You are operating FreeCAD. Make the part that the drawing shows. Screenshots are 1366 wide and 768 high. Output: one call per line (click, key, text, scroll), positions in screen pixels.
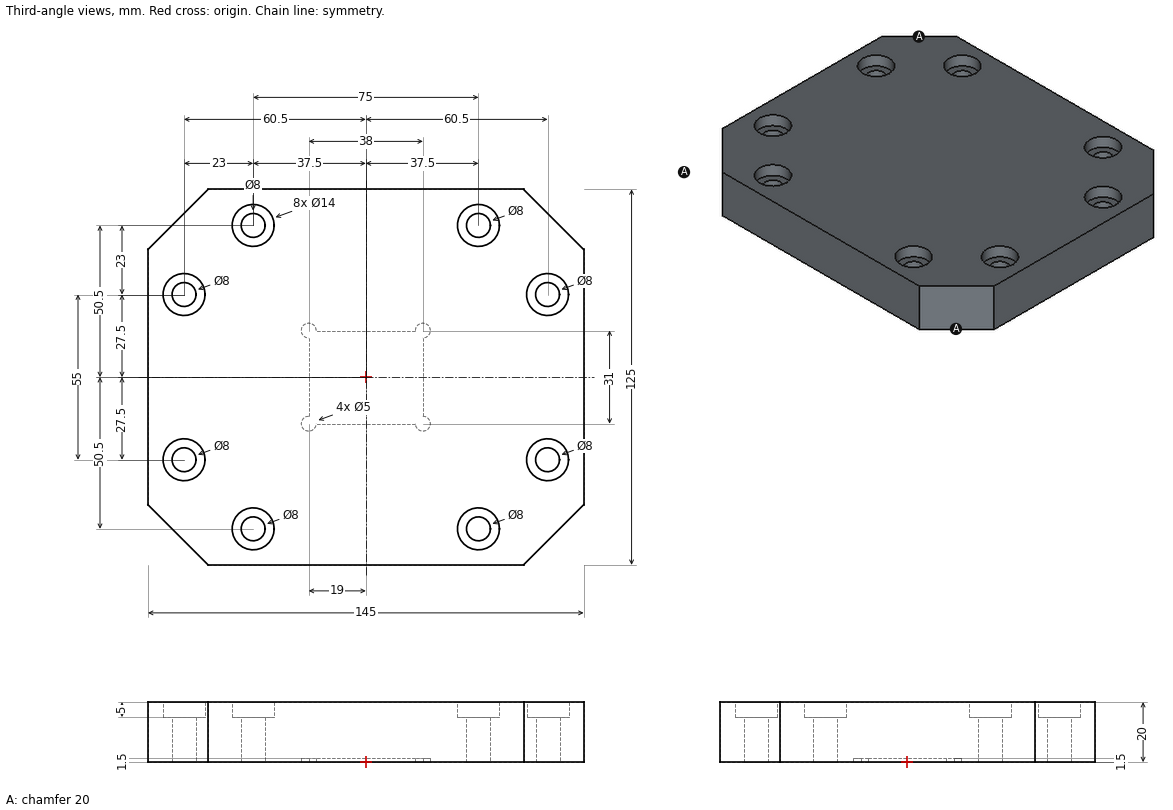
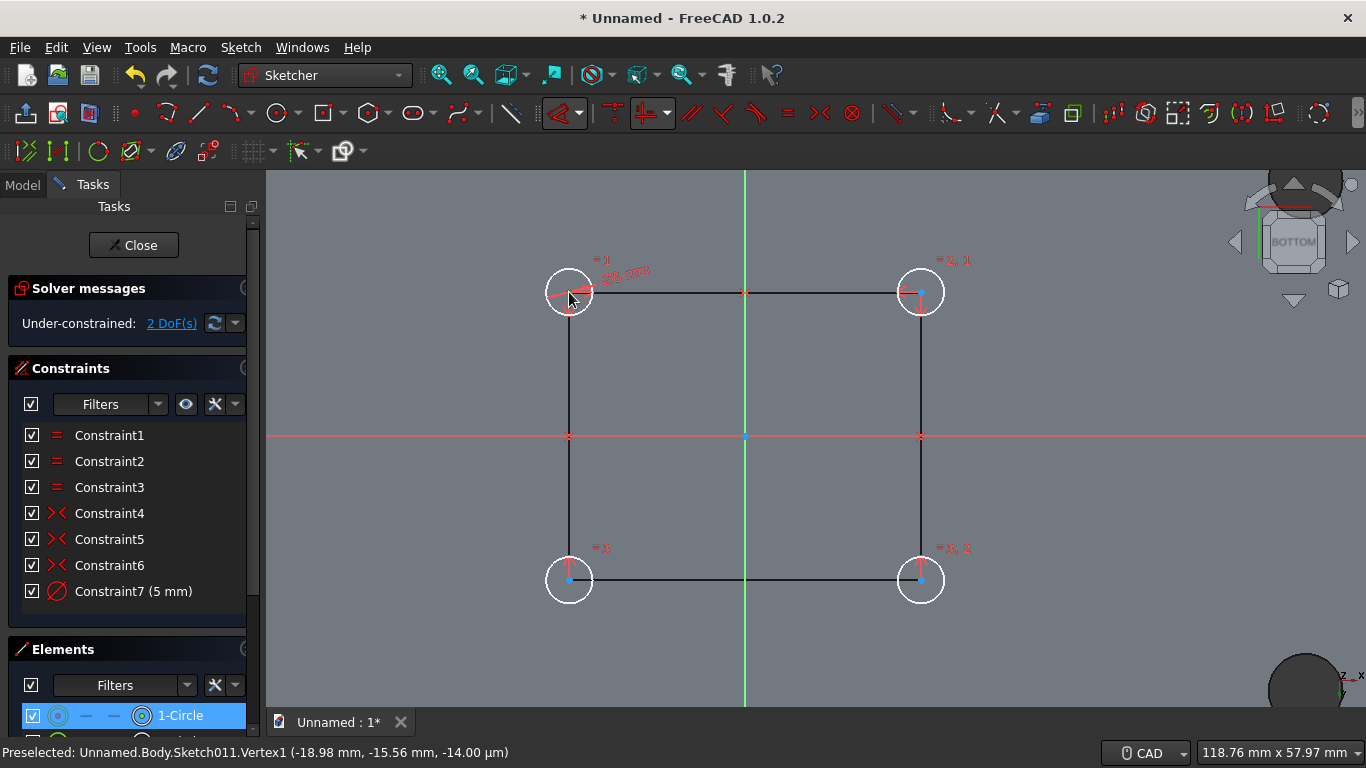
key(l)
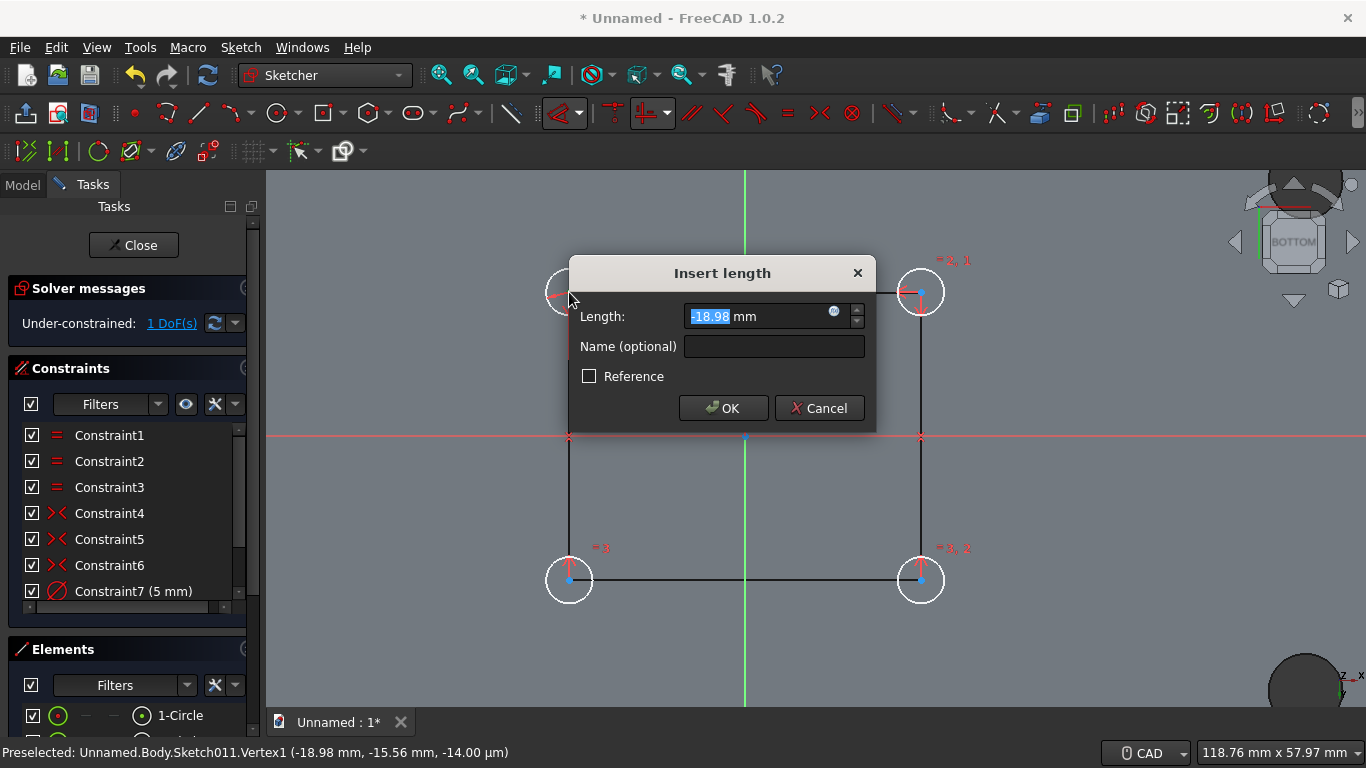
text(-19)
key(Return)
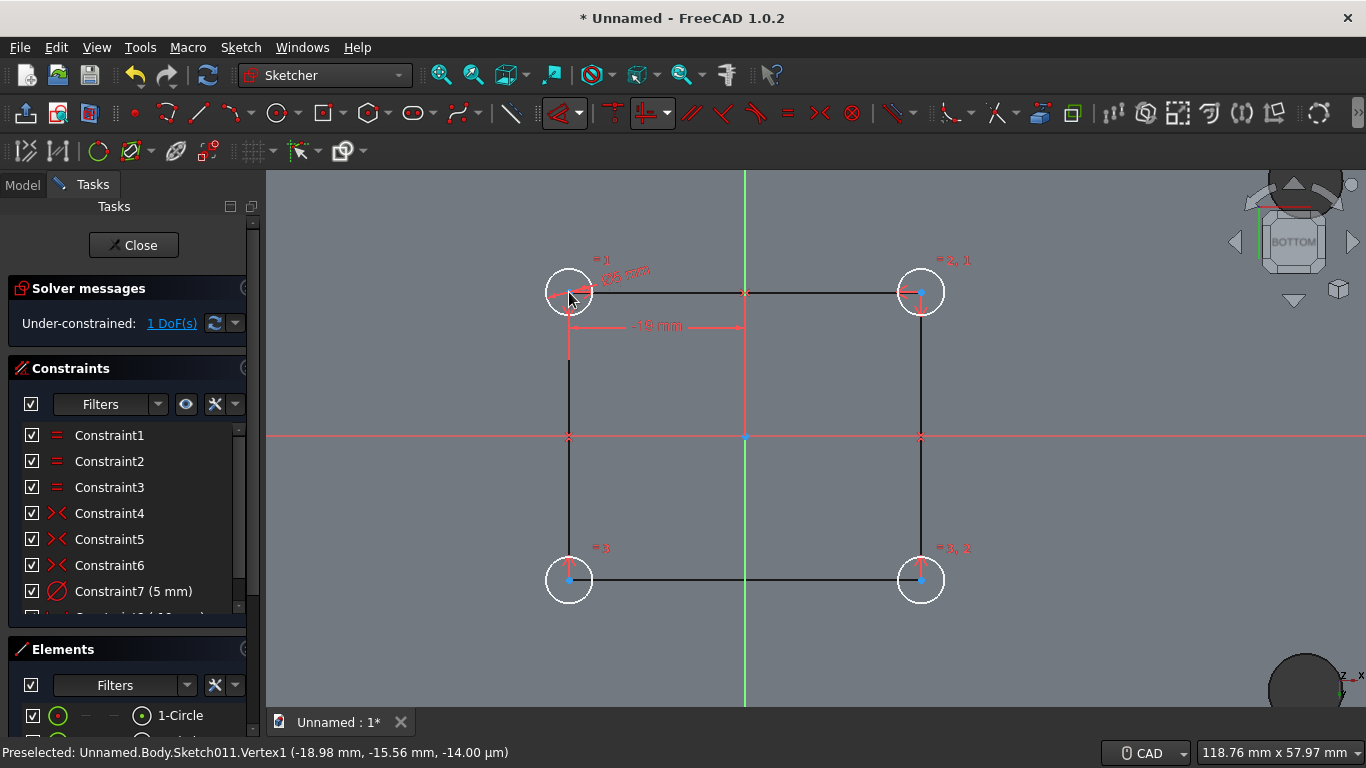
click(921, 292)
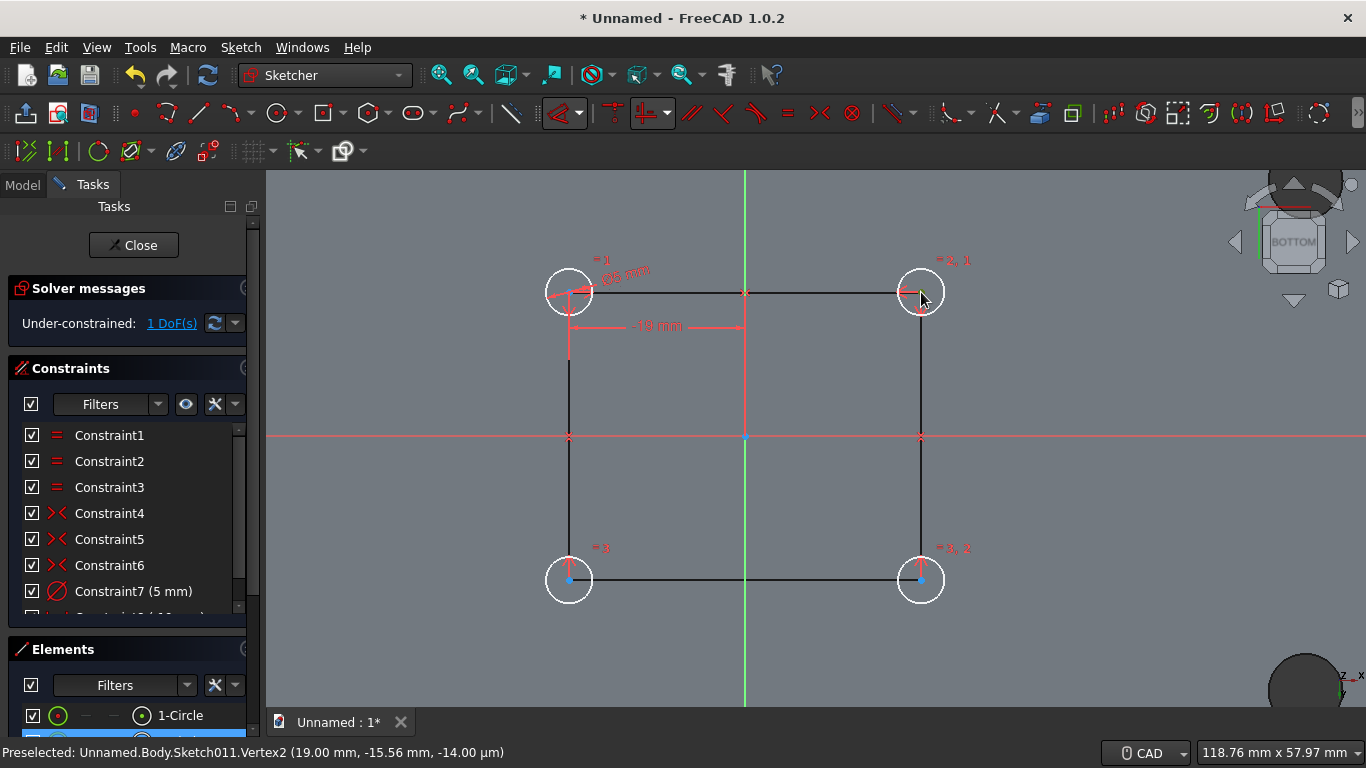
click(921, 580)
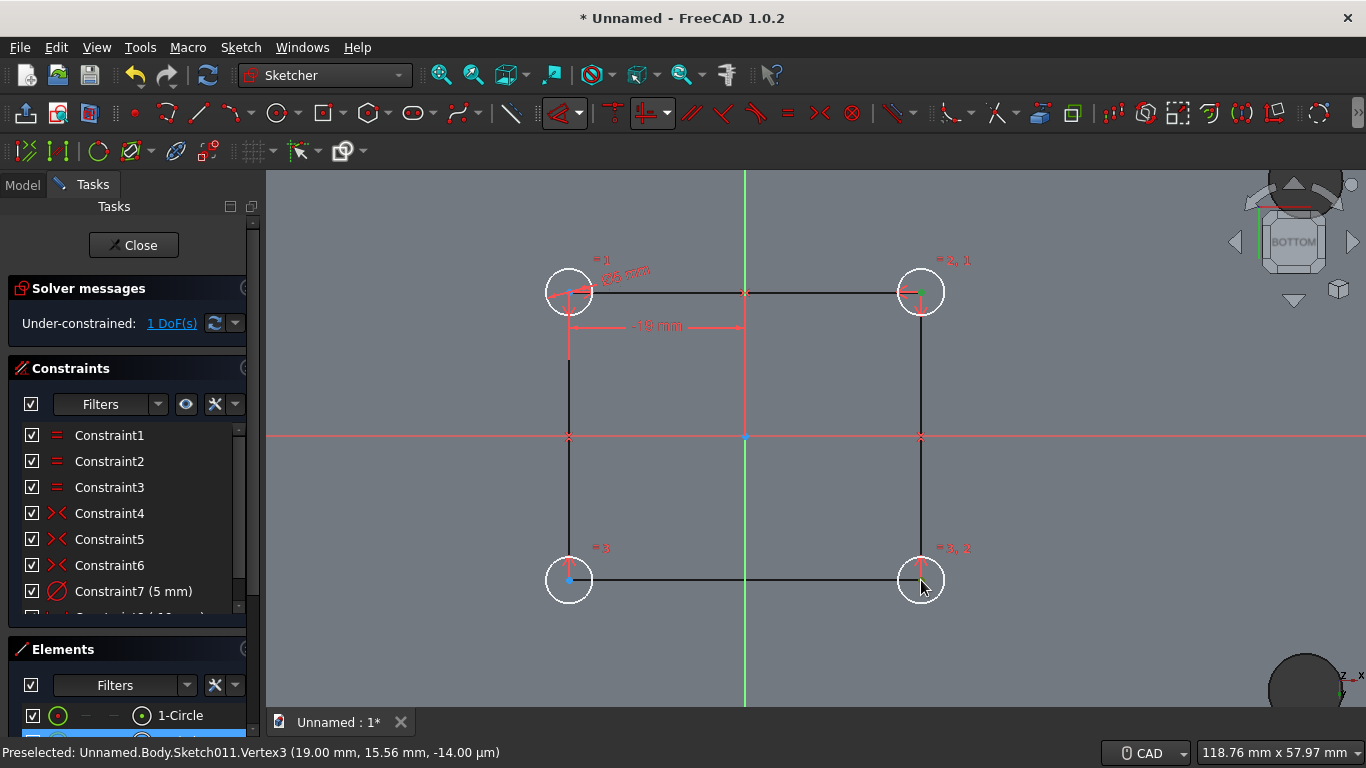
key(i)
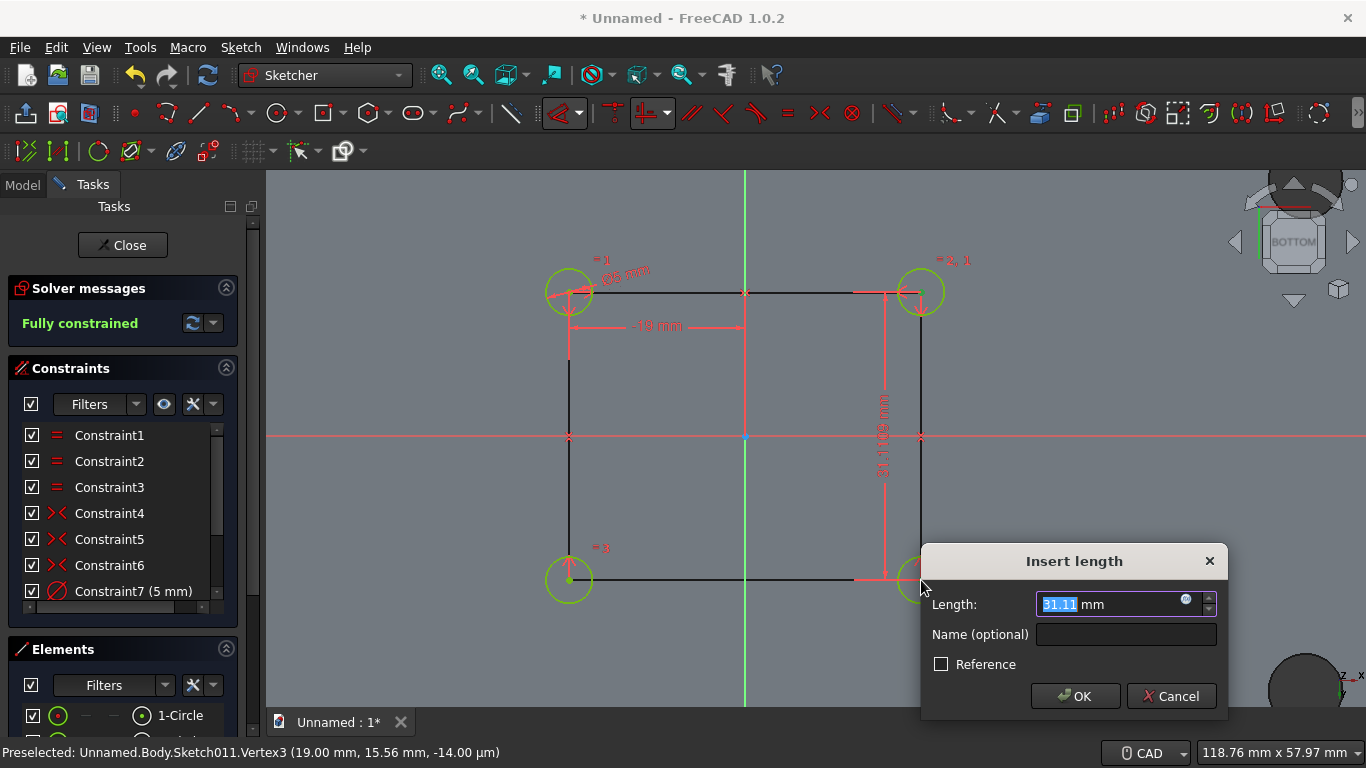
text(31)
key(Return)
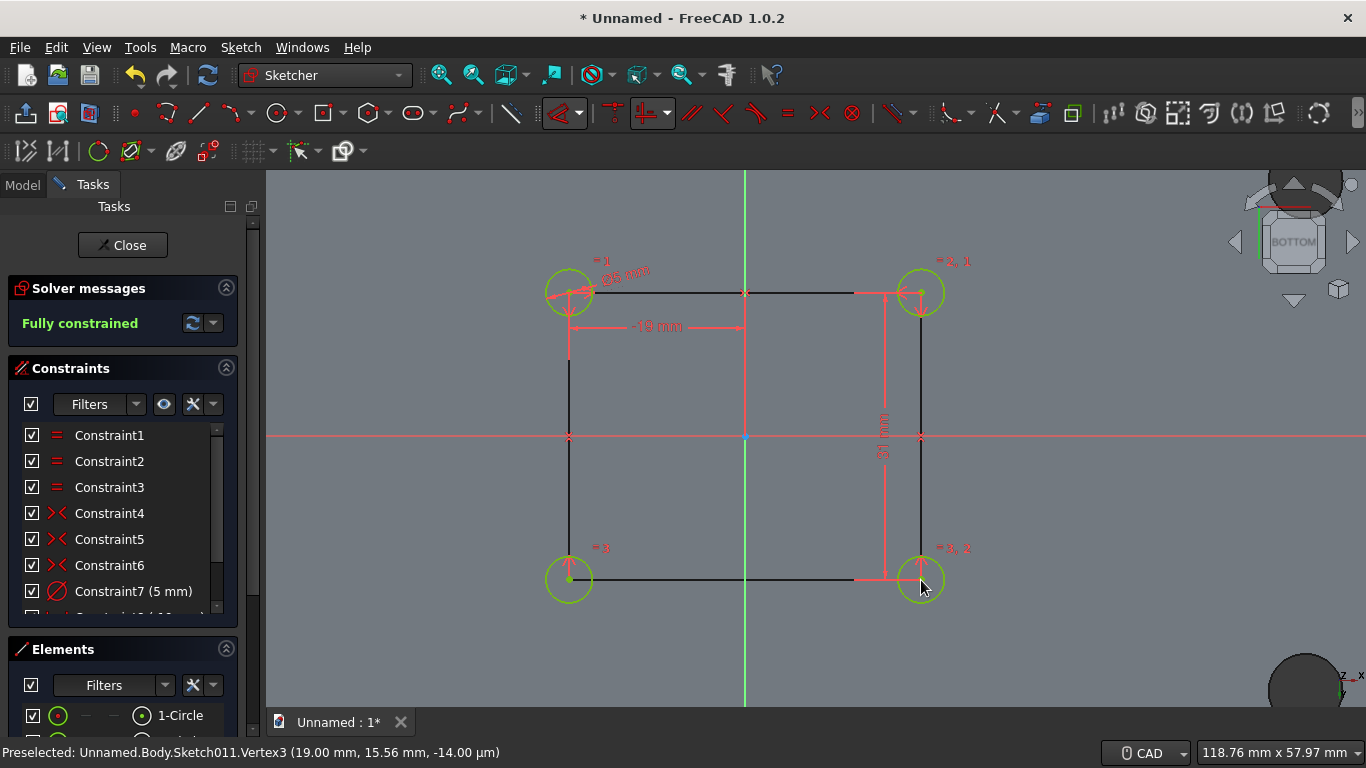
click(123, 245)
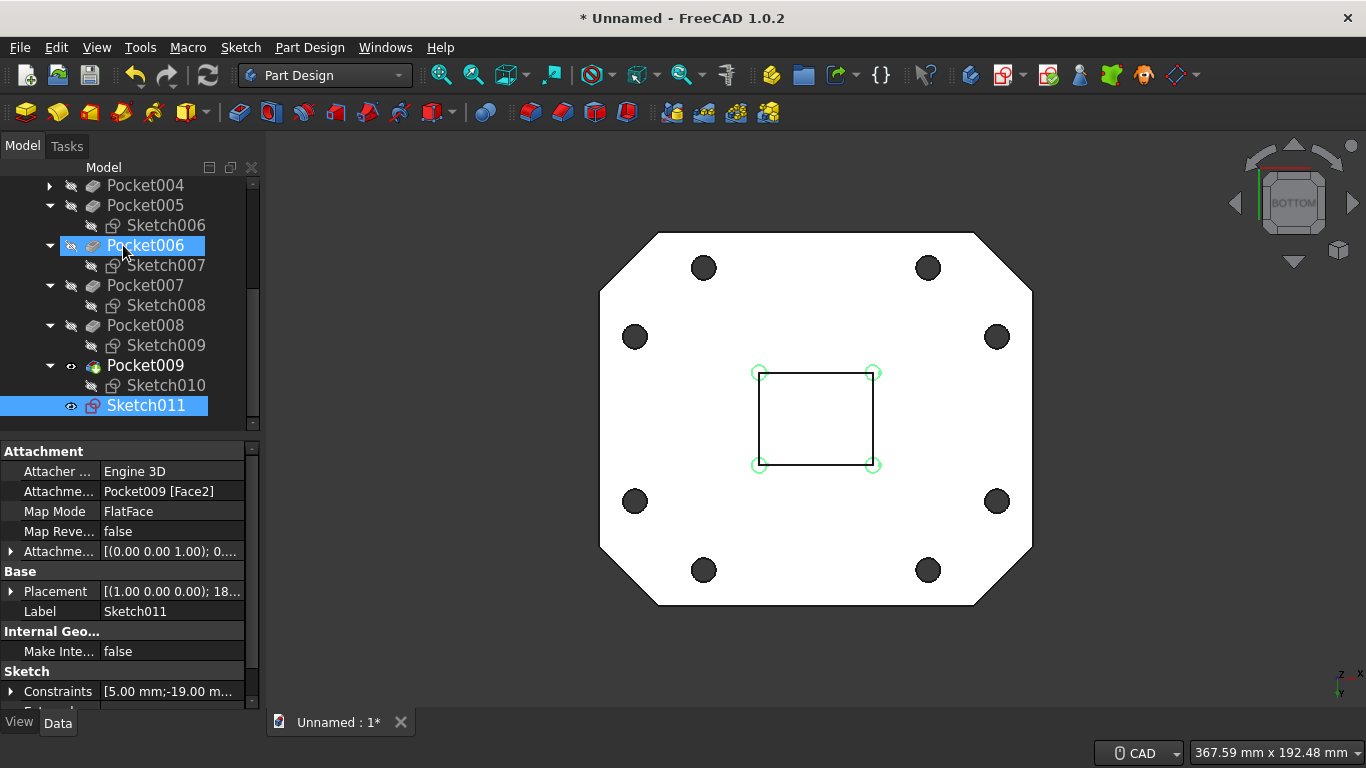
click(240, 112)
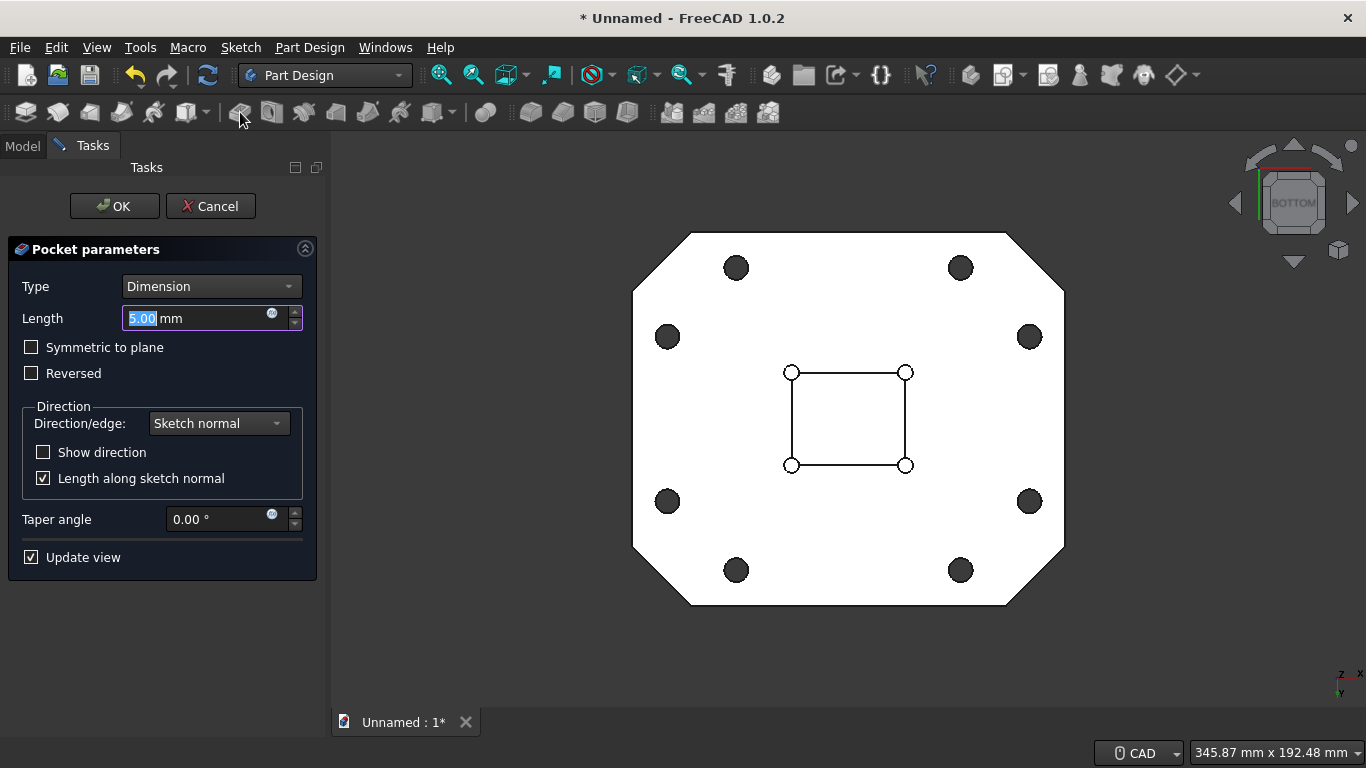
text(1.5)
key(Tab)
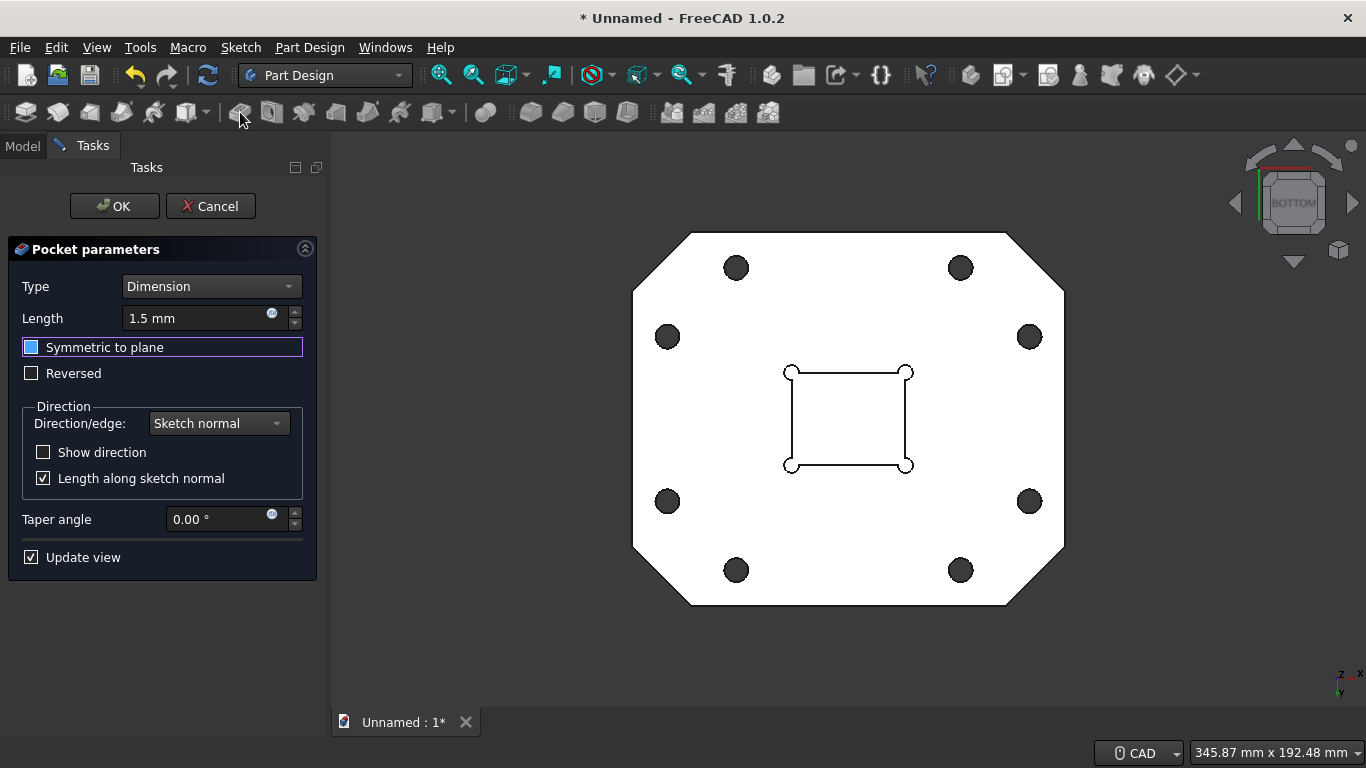
click(115, 206)